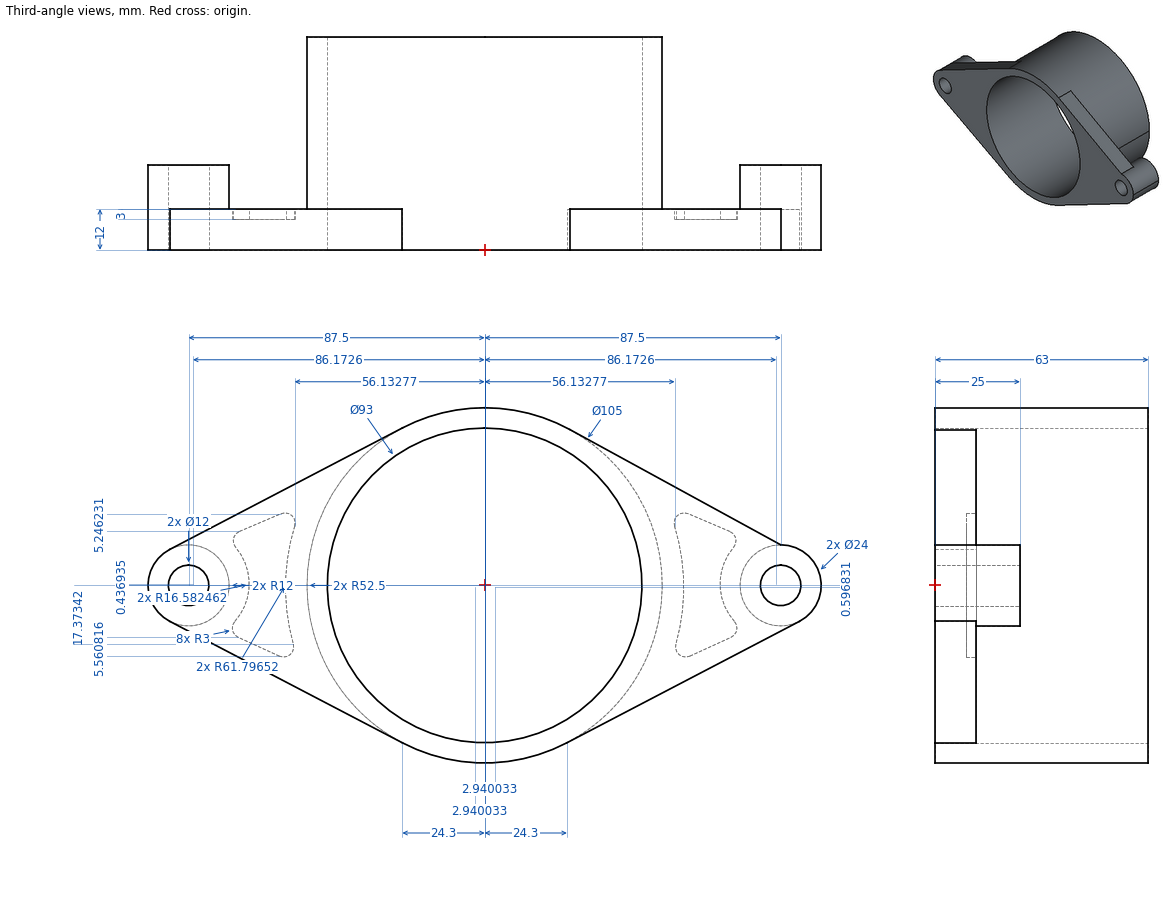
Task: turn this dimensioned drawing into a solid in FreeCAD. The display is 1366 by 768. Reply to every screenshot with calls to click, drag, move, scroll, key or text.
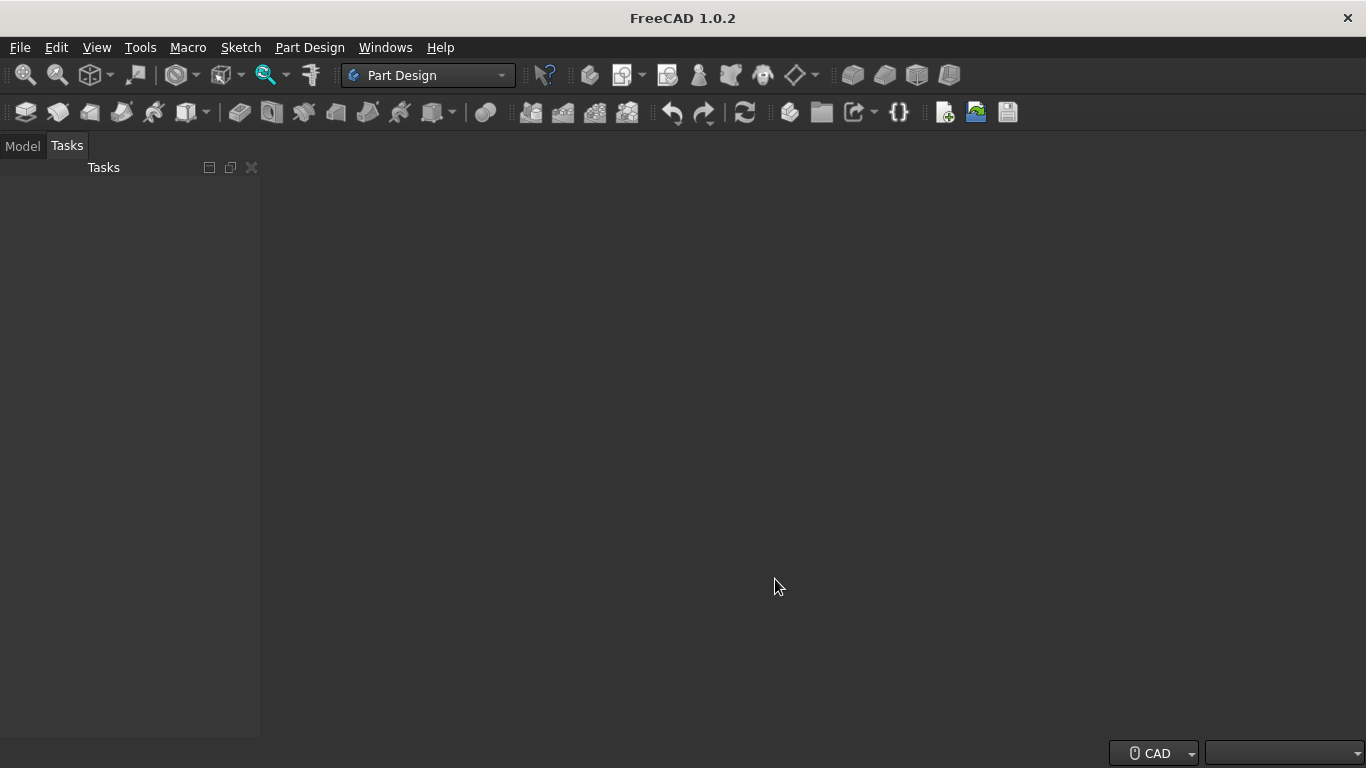
key(ctrl+n)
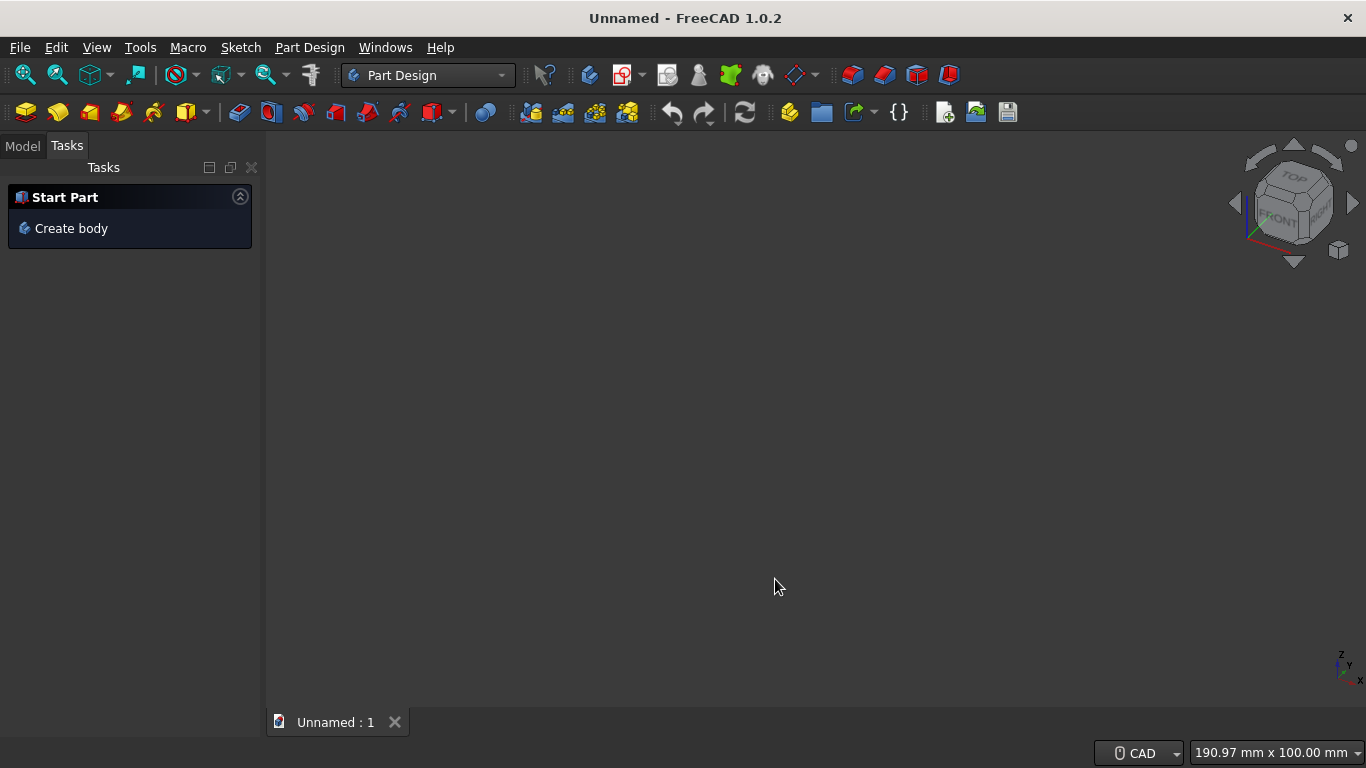
click(622, 76)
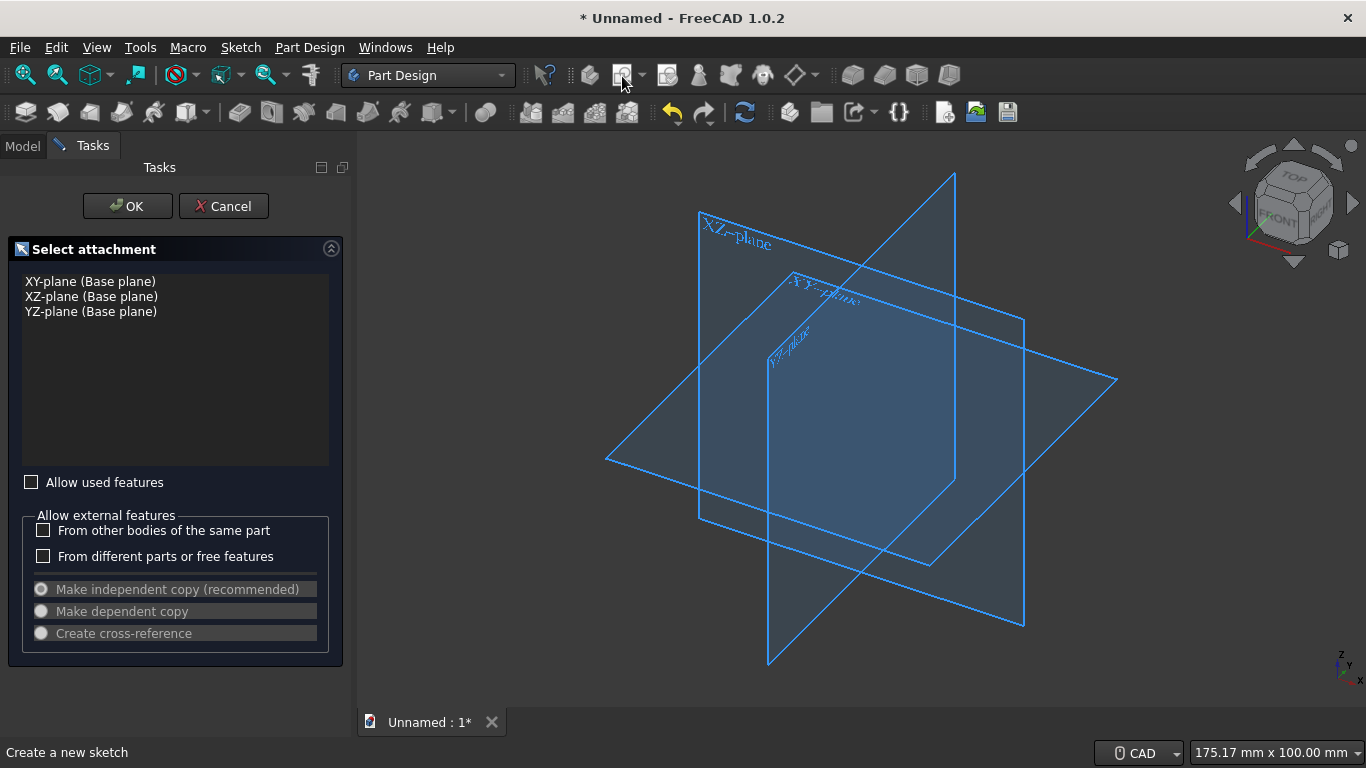
click(82, 296)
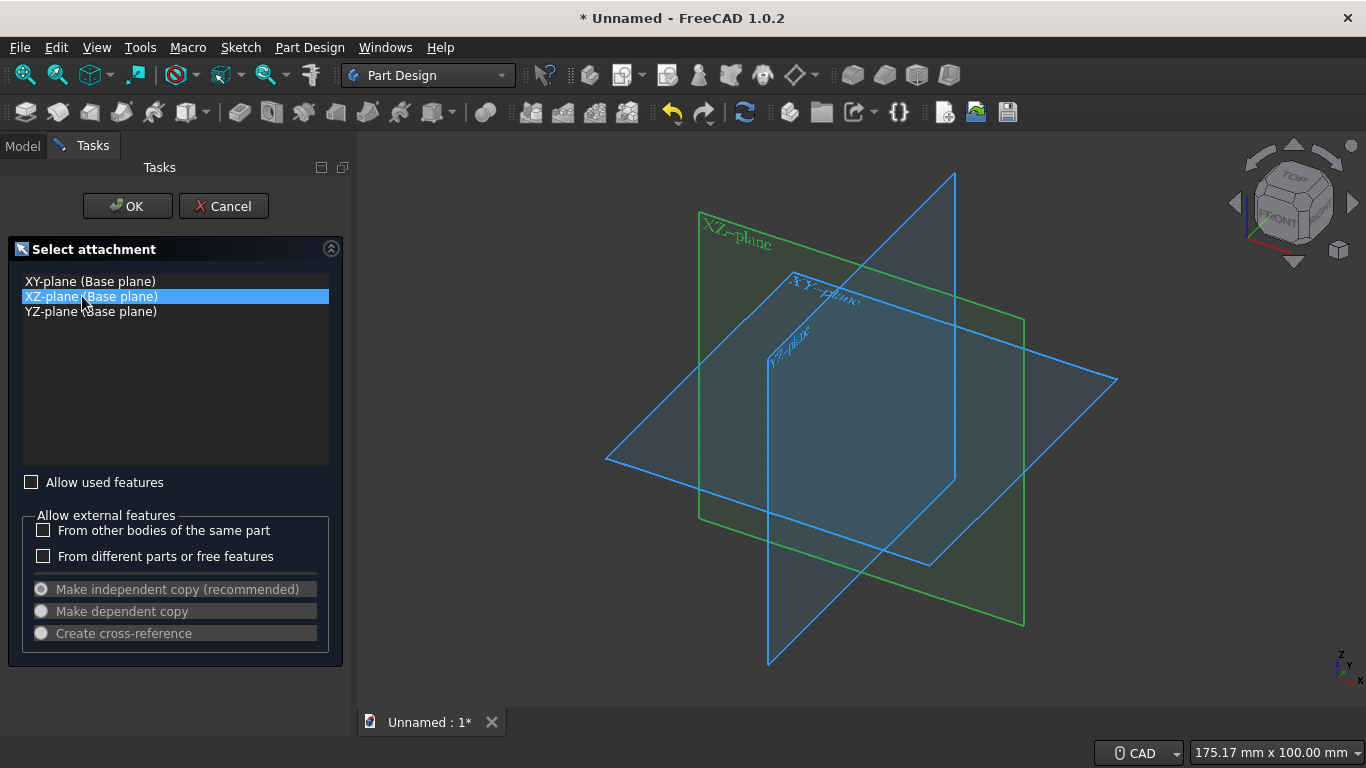
click(128, 206)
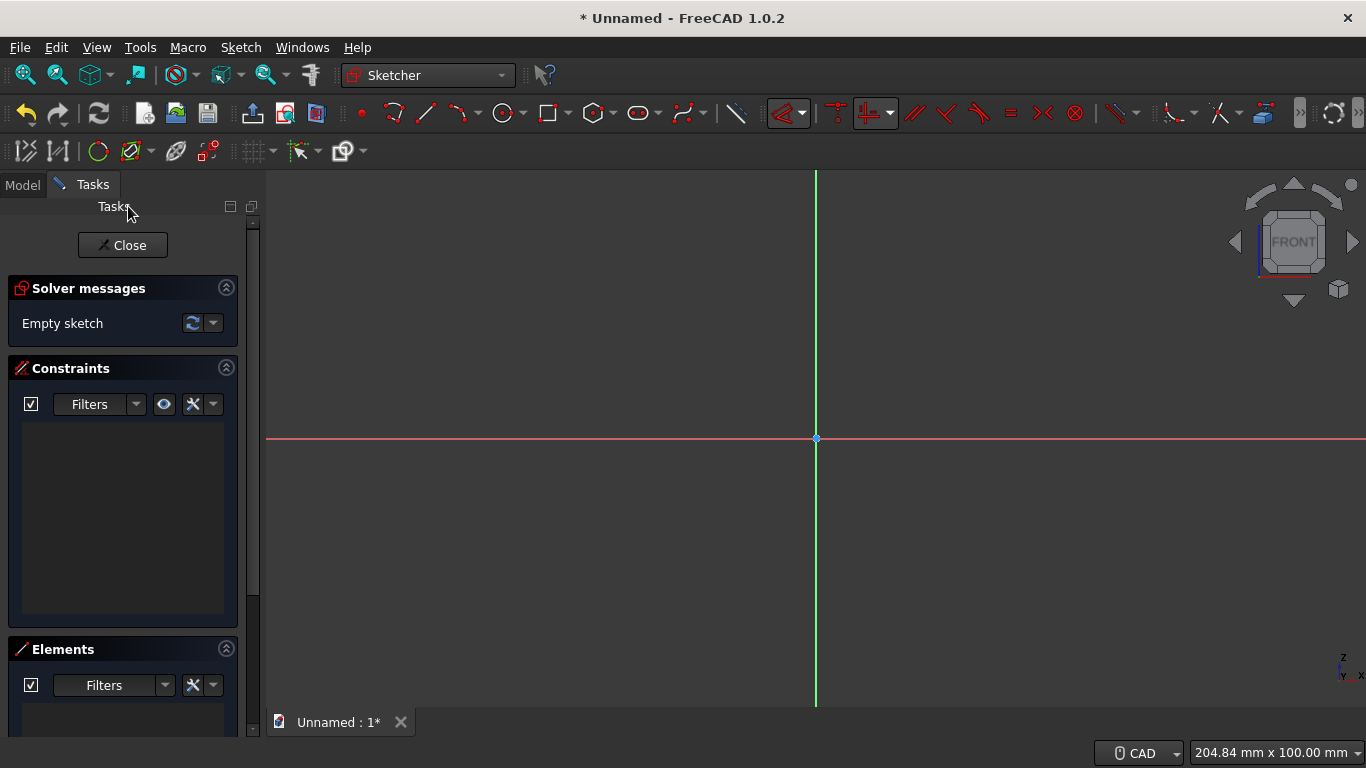
scroll(664, 438, down, 3)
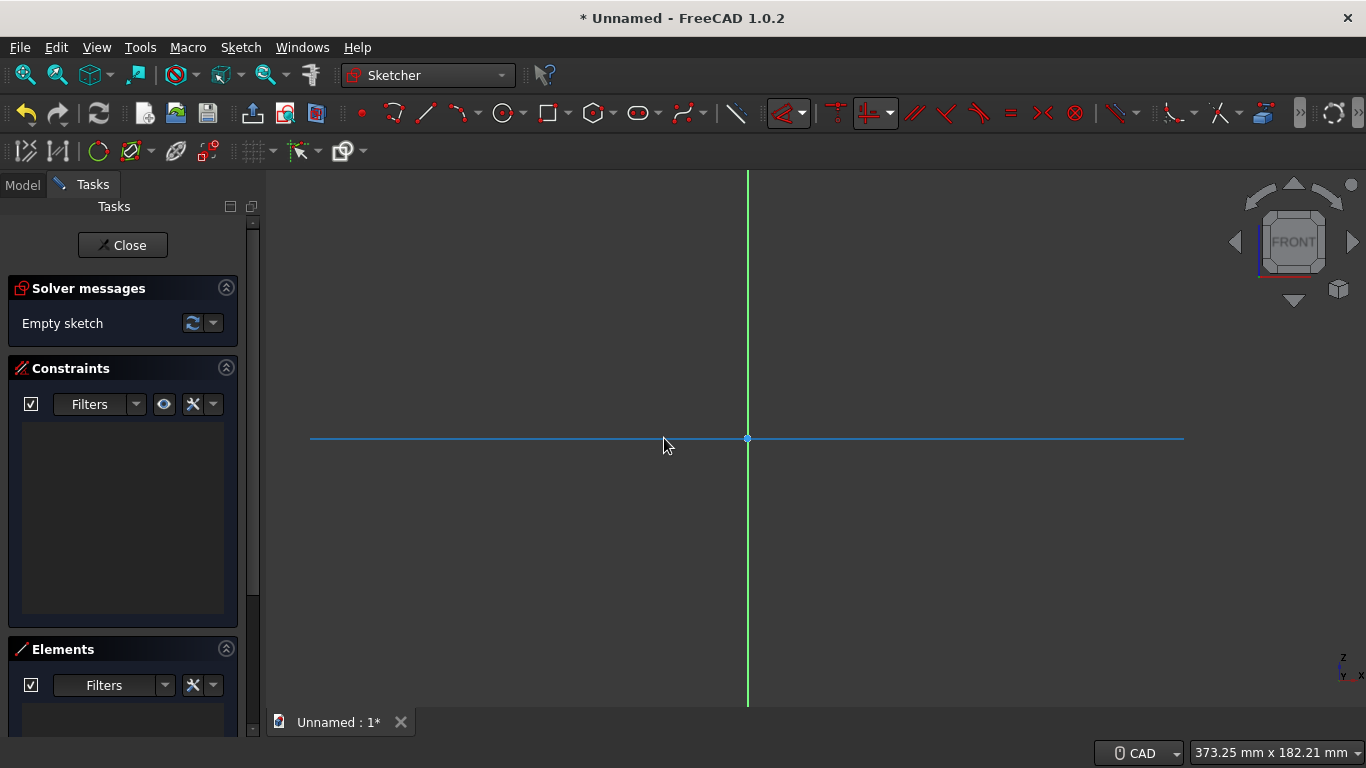
key(g)
key(c)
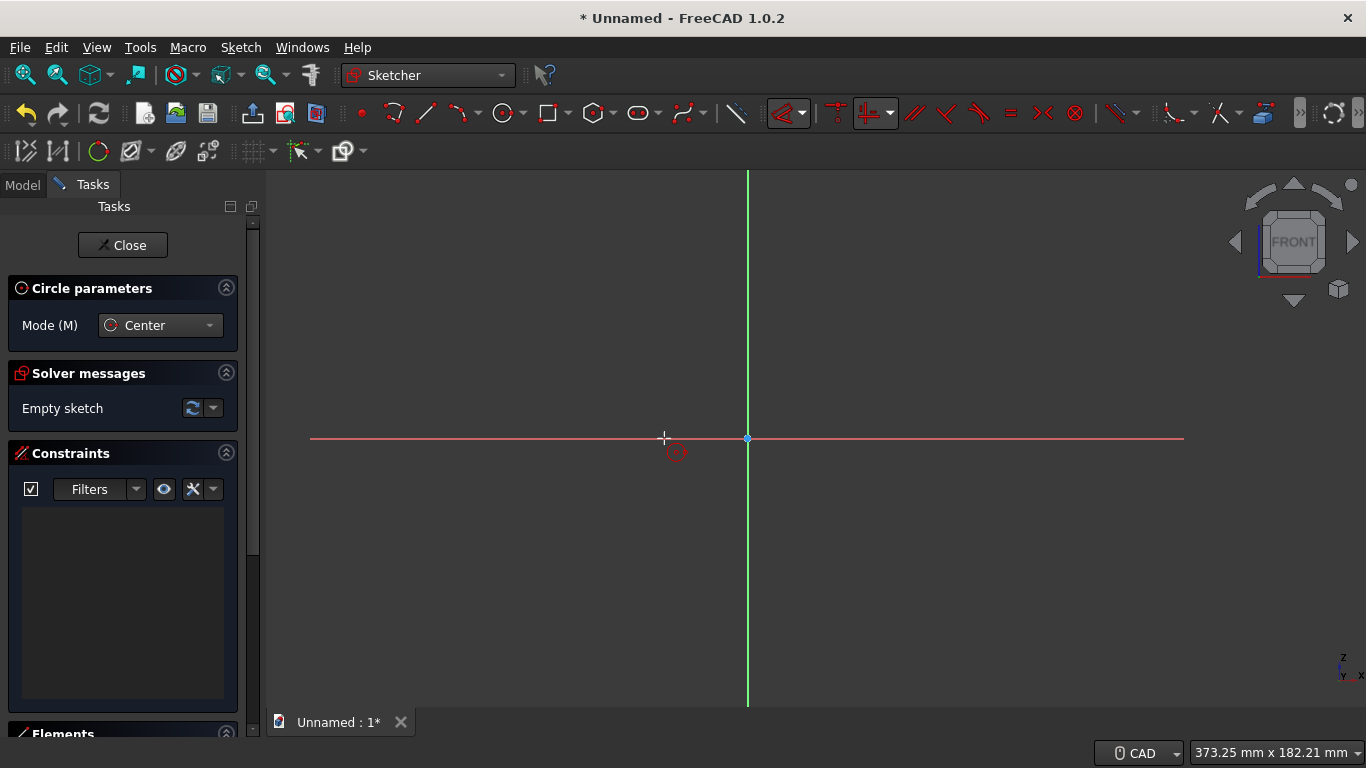
click(748, 438)
move(857, 329)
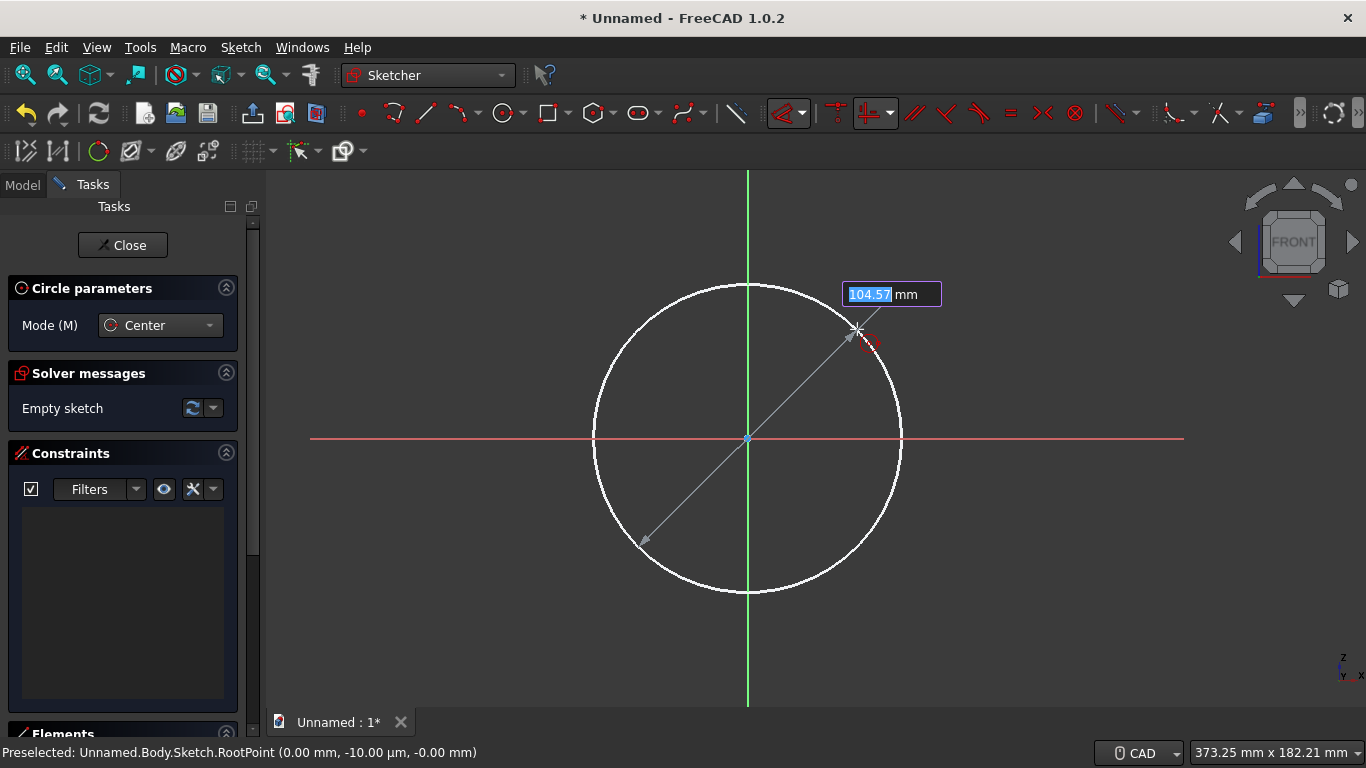
text(105)
key(Return)
key(Escape)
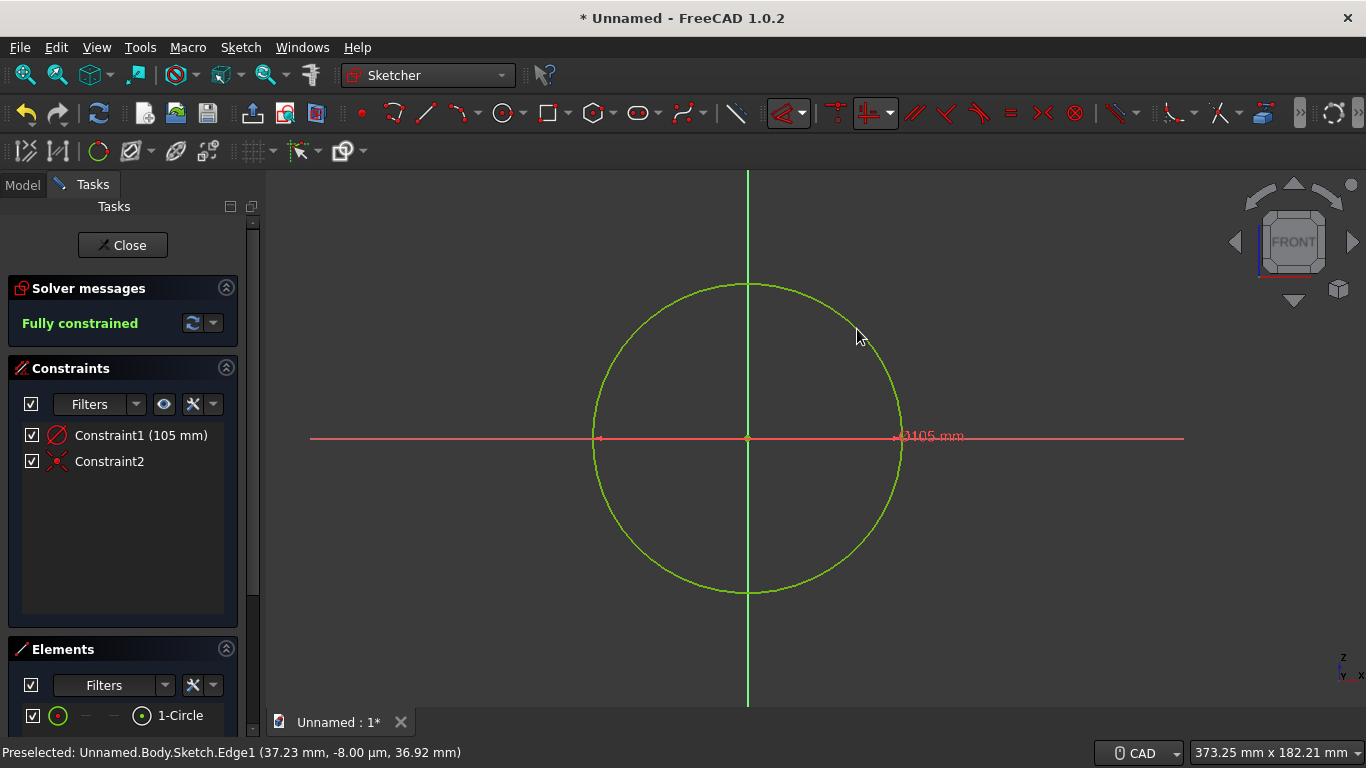
click(123, 245)